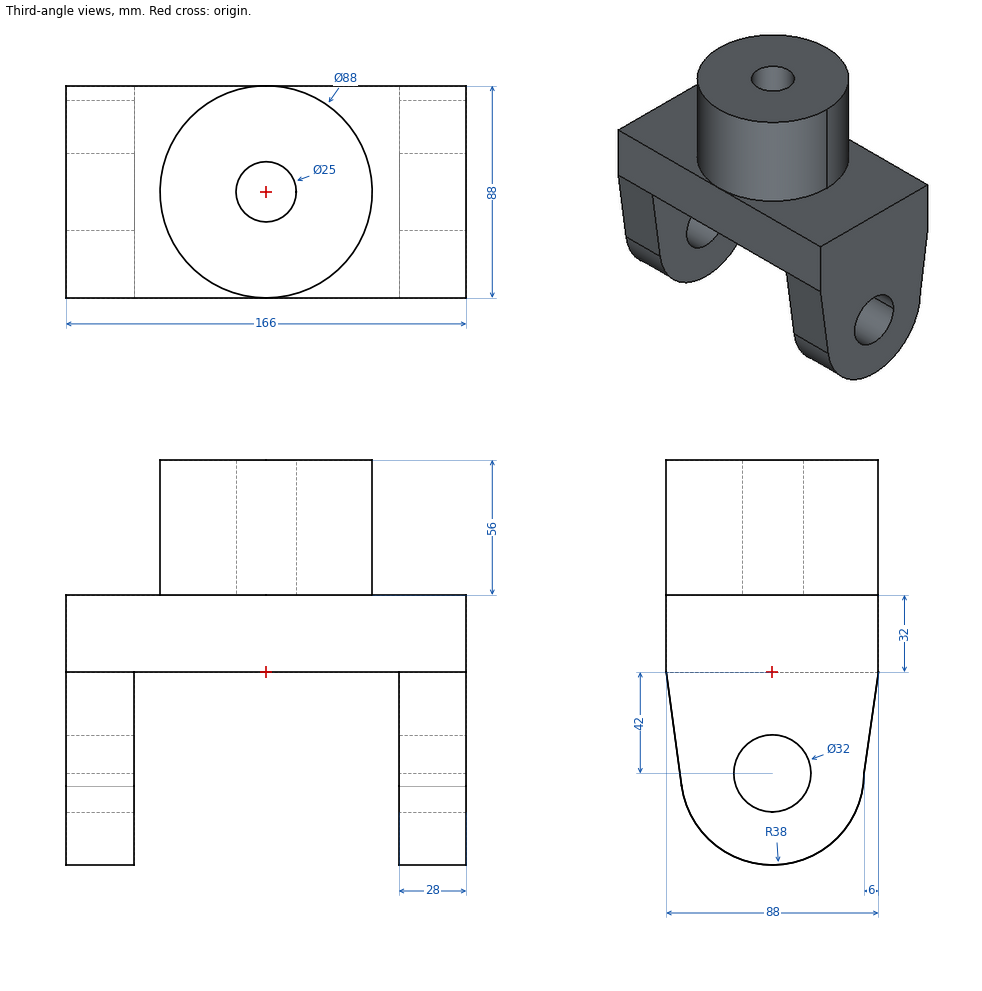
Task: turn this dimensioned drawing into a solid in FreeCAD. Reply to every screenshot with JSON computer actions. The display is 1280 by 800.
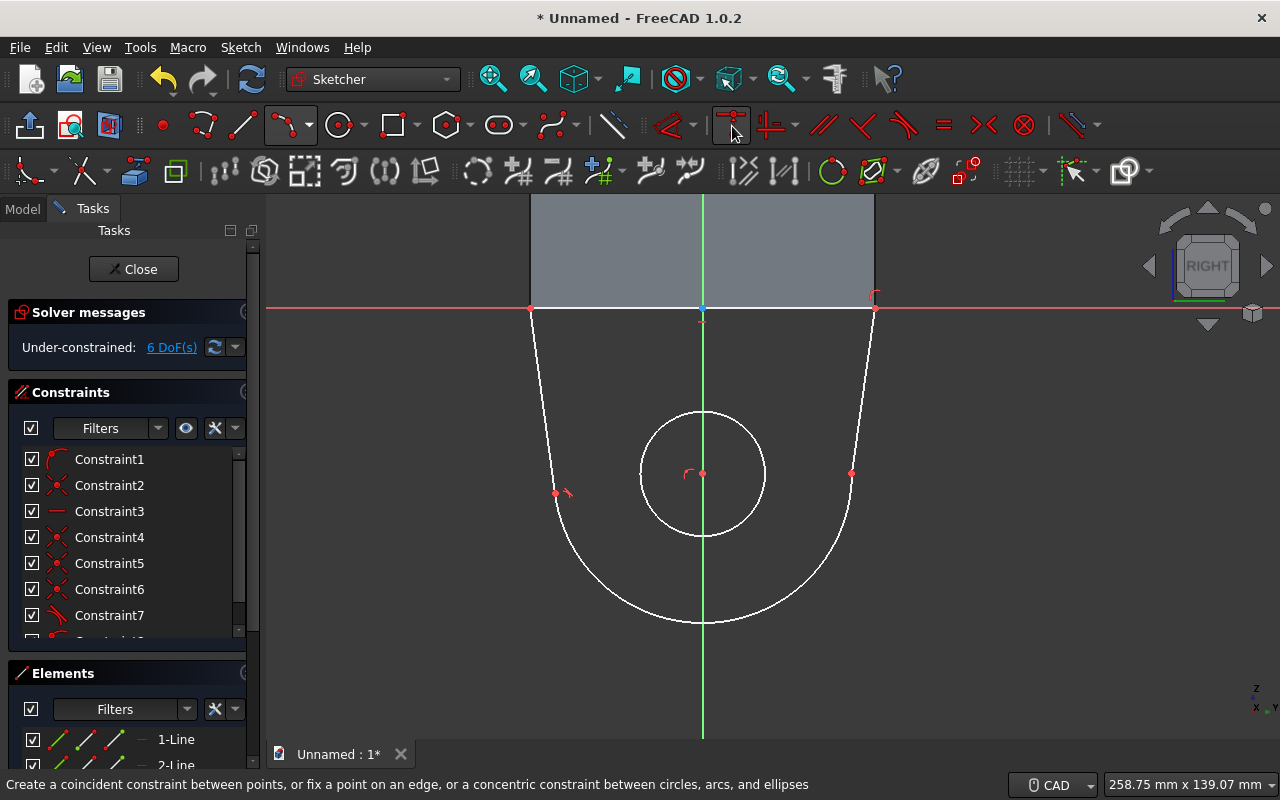
{"action": "left_click", "coordinate": [668, 126]}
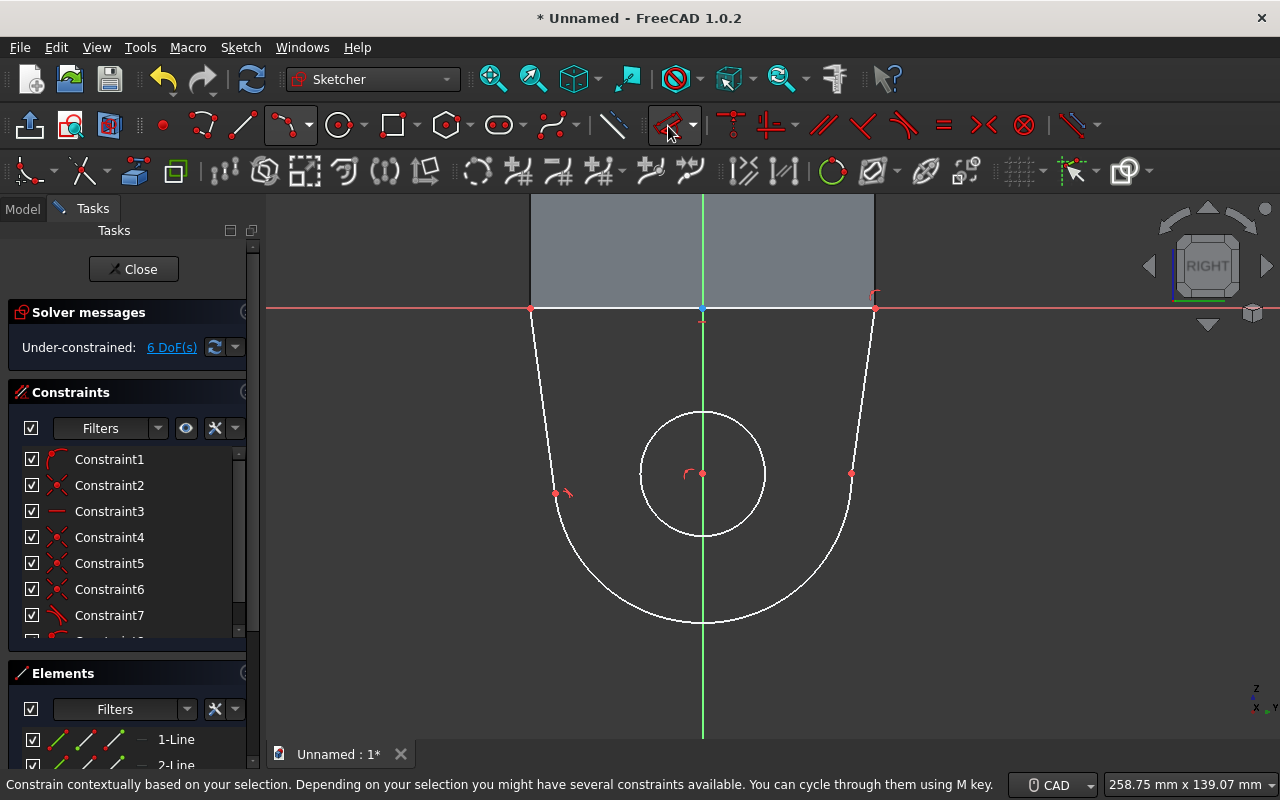
{"action": "left_click", "coordinate": [627, 602]}
{"action": "left_click", "coordinate": [611, 630]}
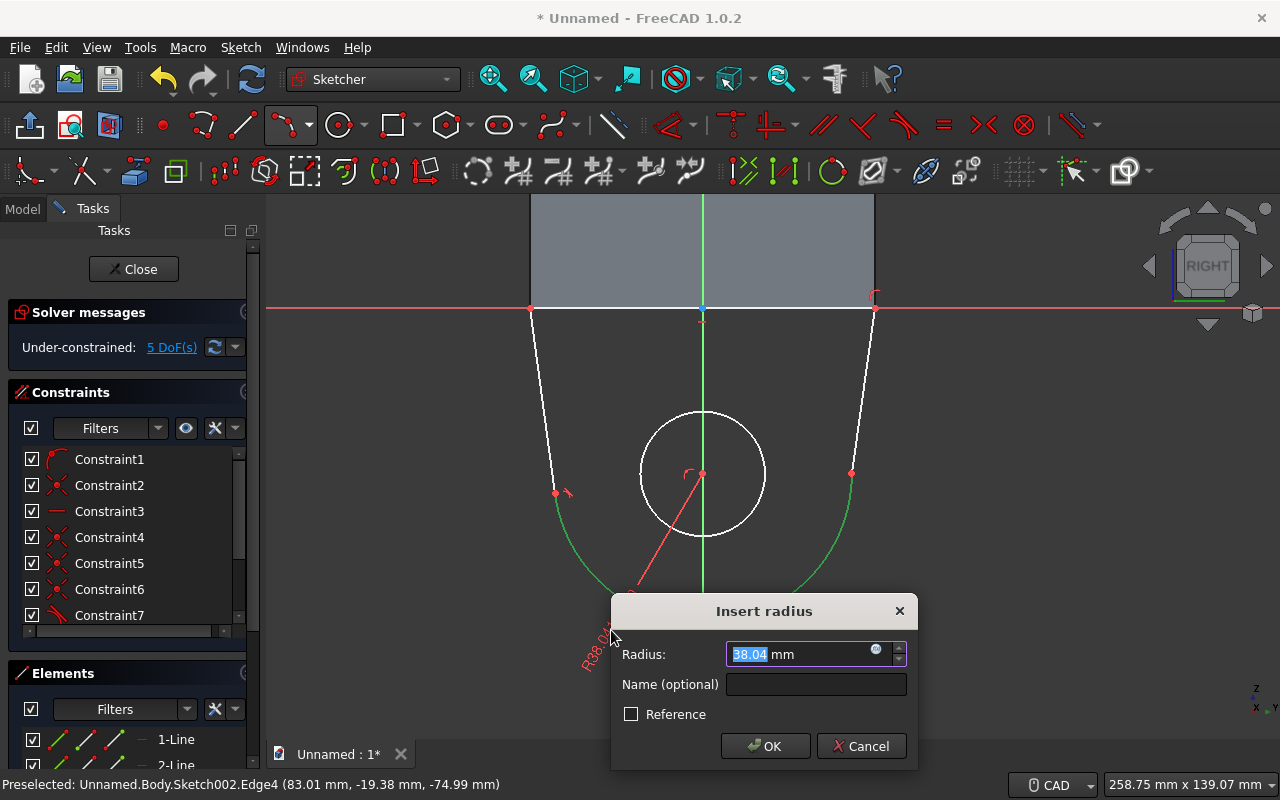
{"action": "type", "text": "38"}
{"action": "key", "text": "Return"}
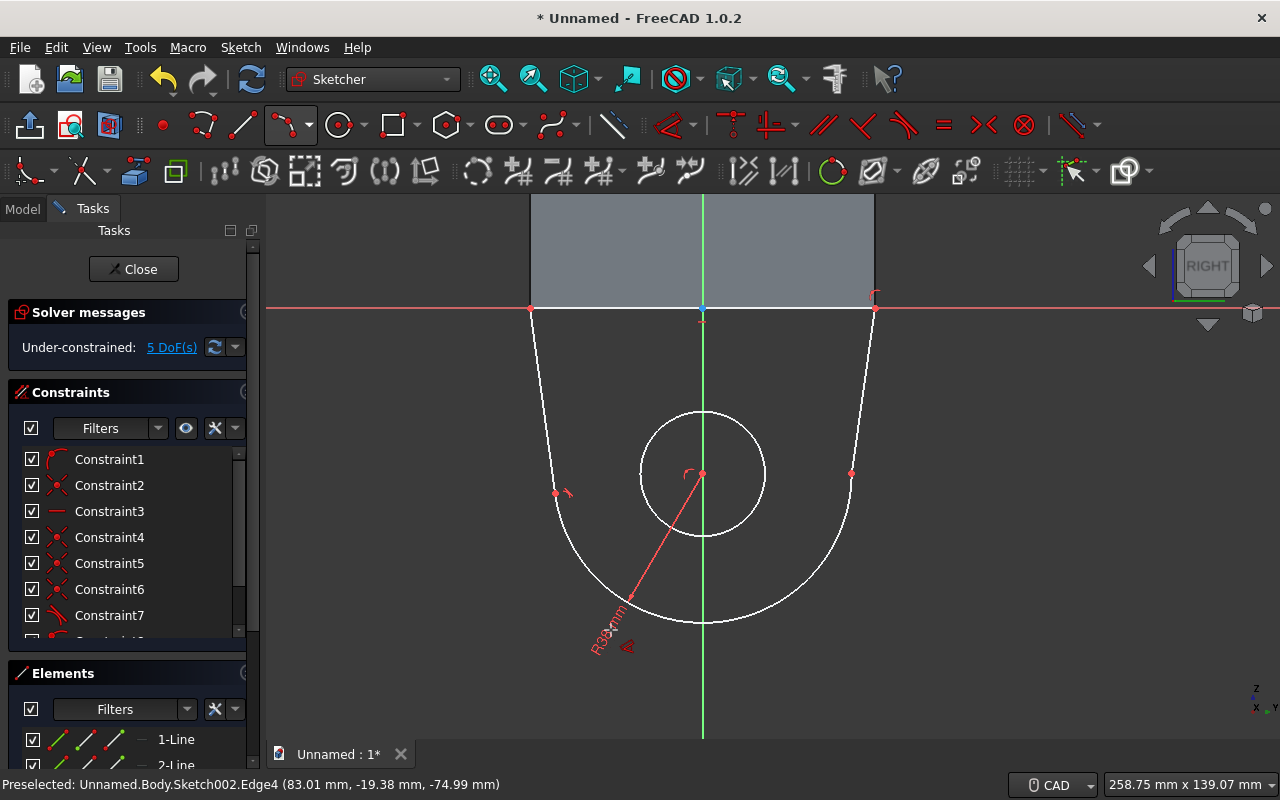
{"action": "left_click", "coordinate": [747, 430]}
{"action": "left_click", "coordinate": [770, 407]}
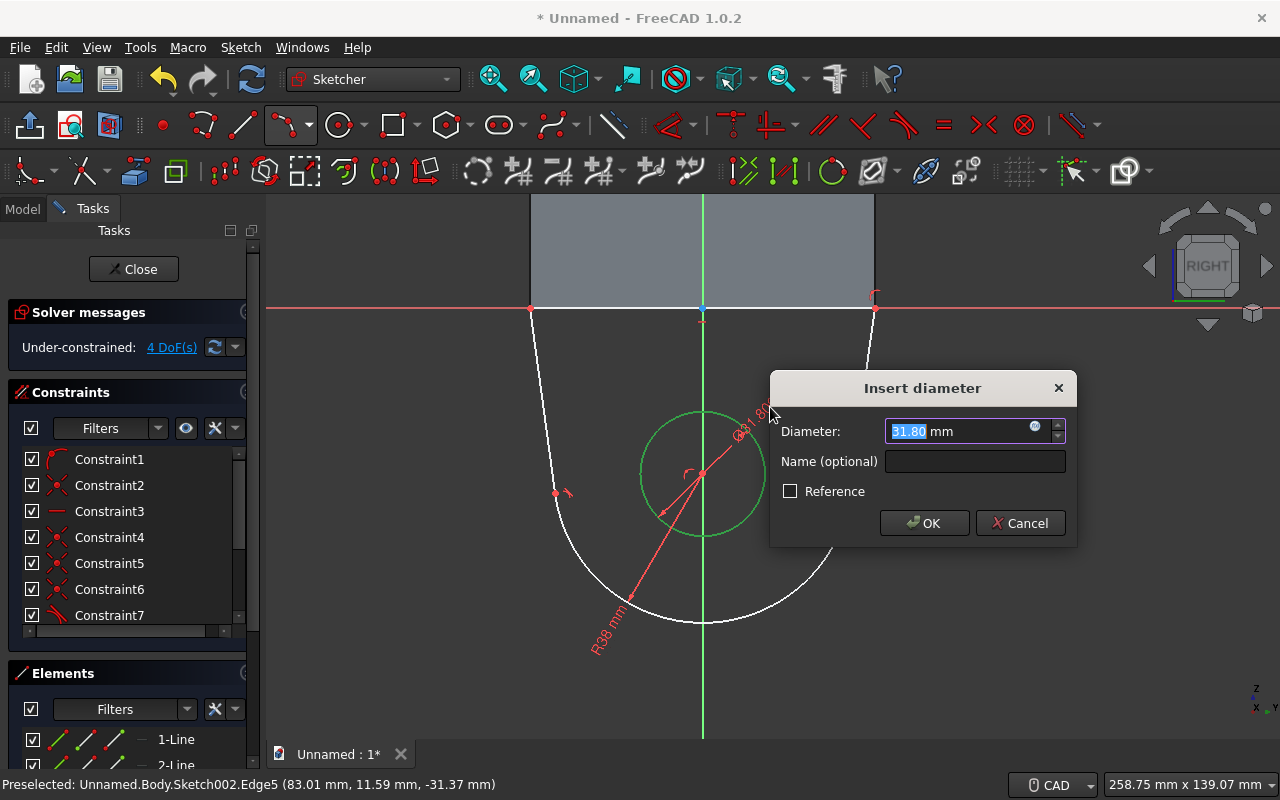
{"action": "type", "text": "32"}
{"action": "key", "text": "Return"}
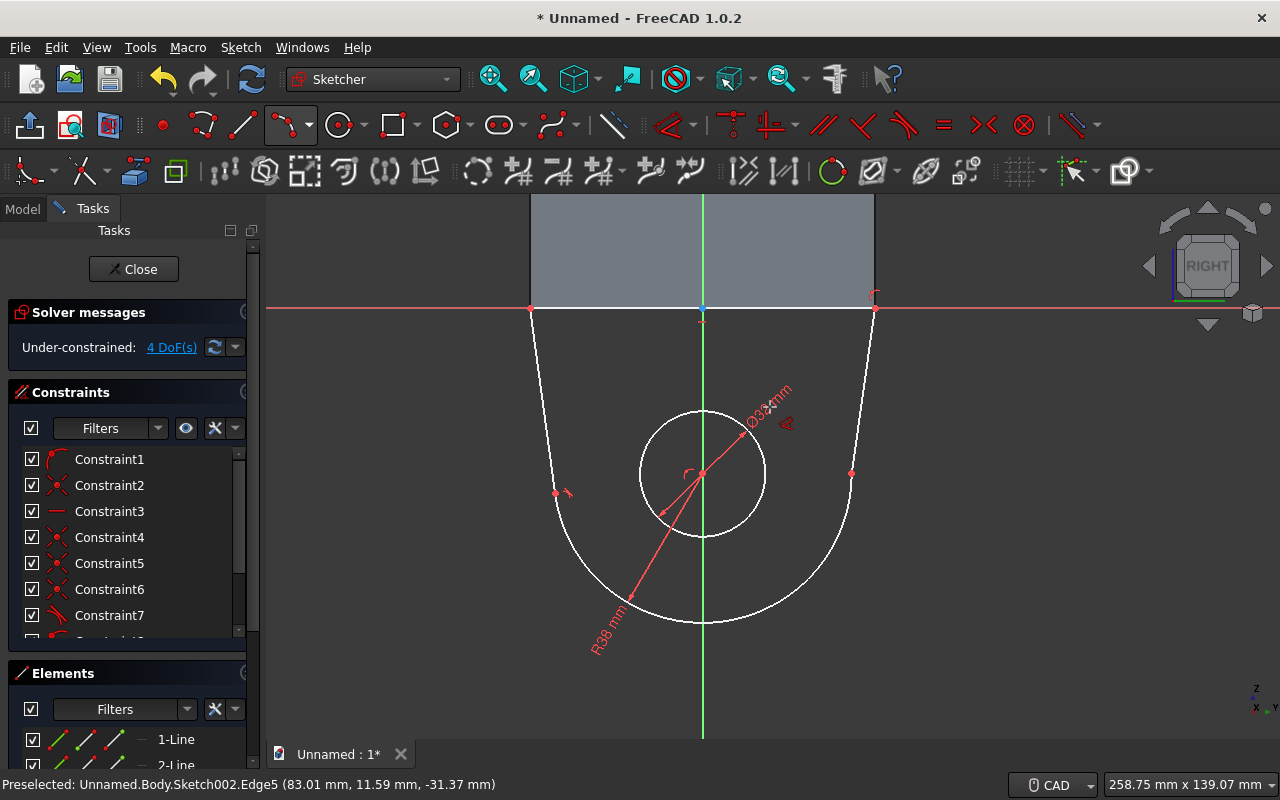
{"action": "left_click", "coordinate": [771, 308]}
{"action": "left_click", "coordinate": [623, 274]}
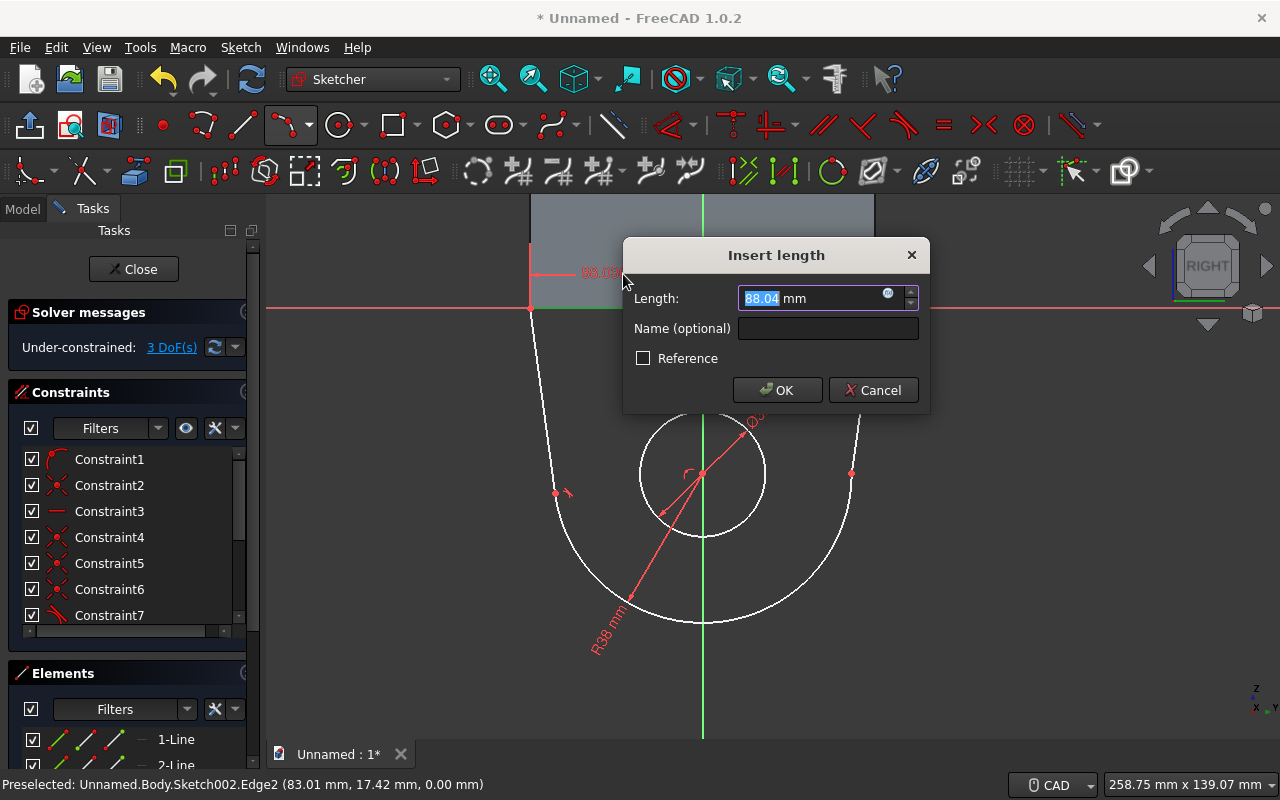
{"action": "type", "text": "88"}
{"action": "key", "text": "Return"}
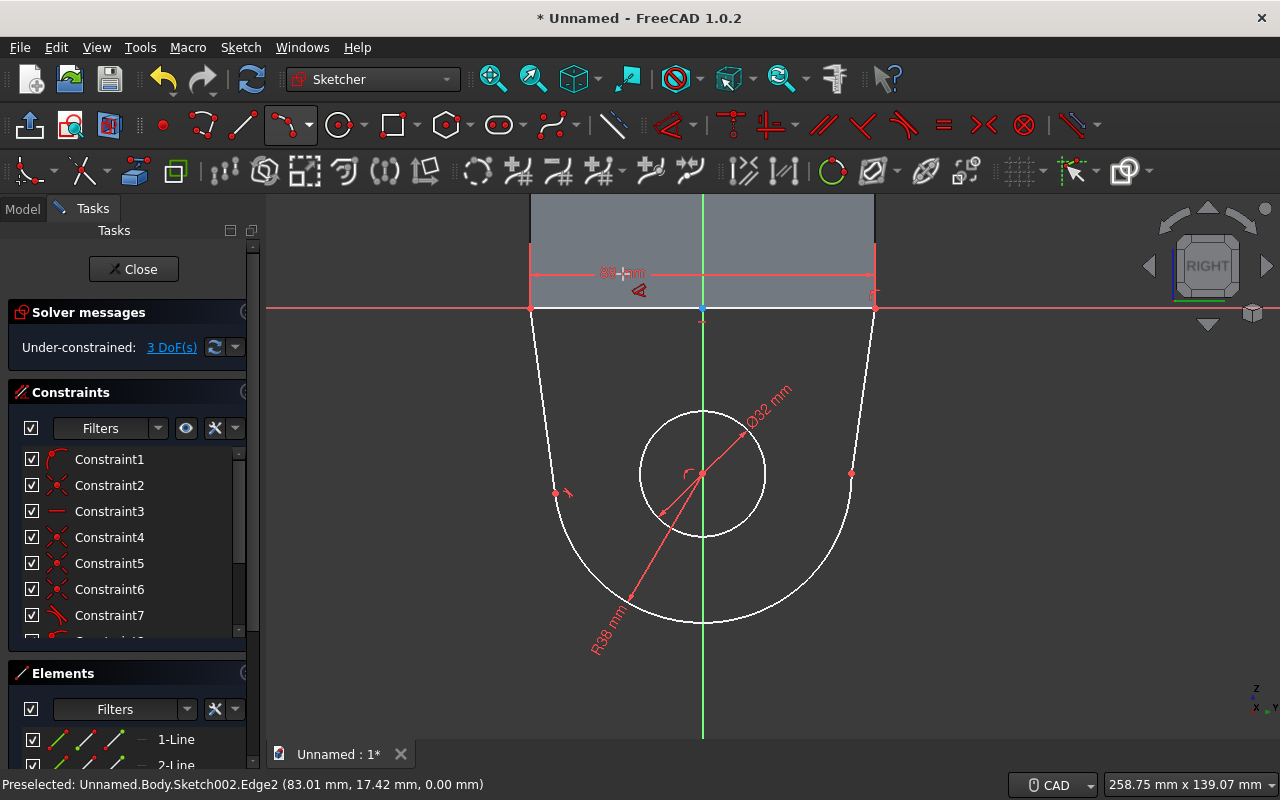
{"action": "scroll", "coordinate": [859, 424], "scroll_direction": "up", "scroll_amount": 3}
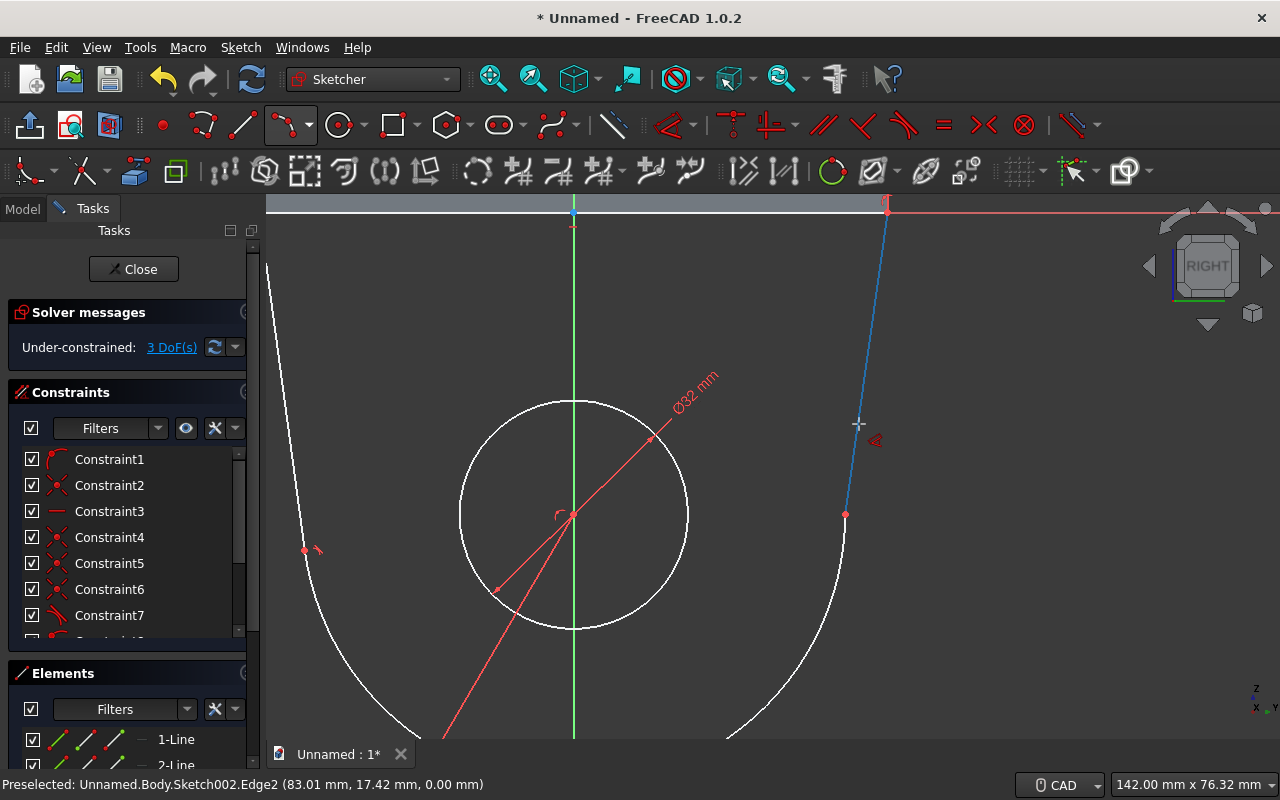
{"action": "left_click", "coordinate": [858, 424]}
{"action": "left_click", "coordinate": [866, 549]}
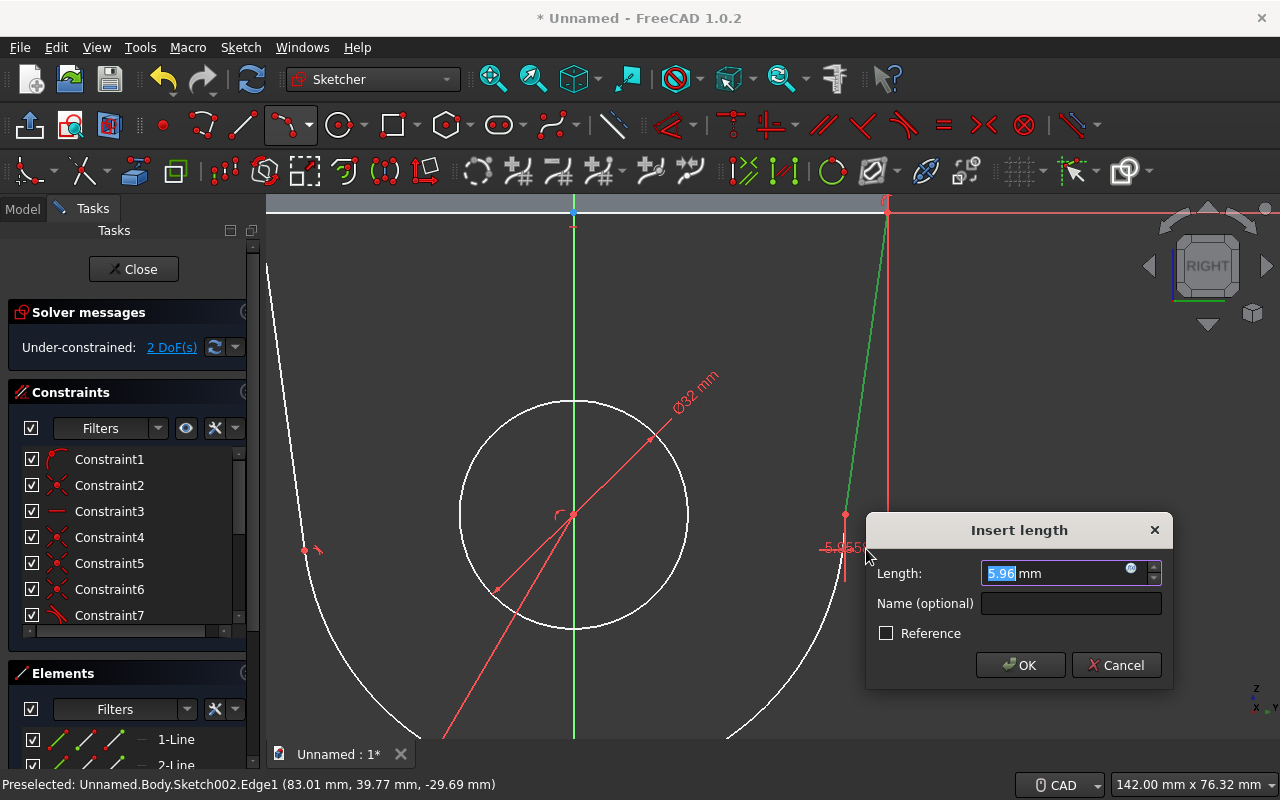
{"action": "type", "text": "6"}
{"action": "key", "text": "Return"}